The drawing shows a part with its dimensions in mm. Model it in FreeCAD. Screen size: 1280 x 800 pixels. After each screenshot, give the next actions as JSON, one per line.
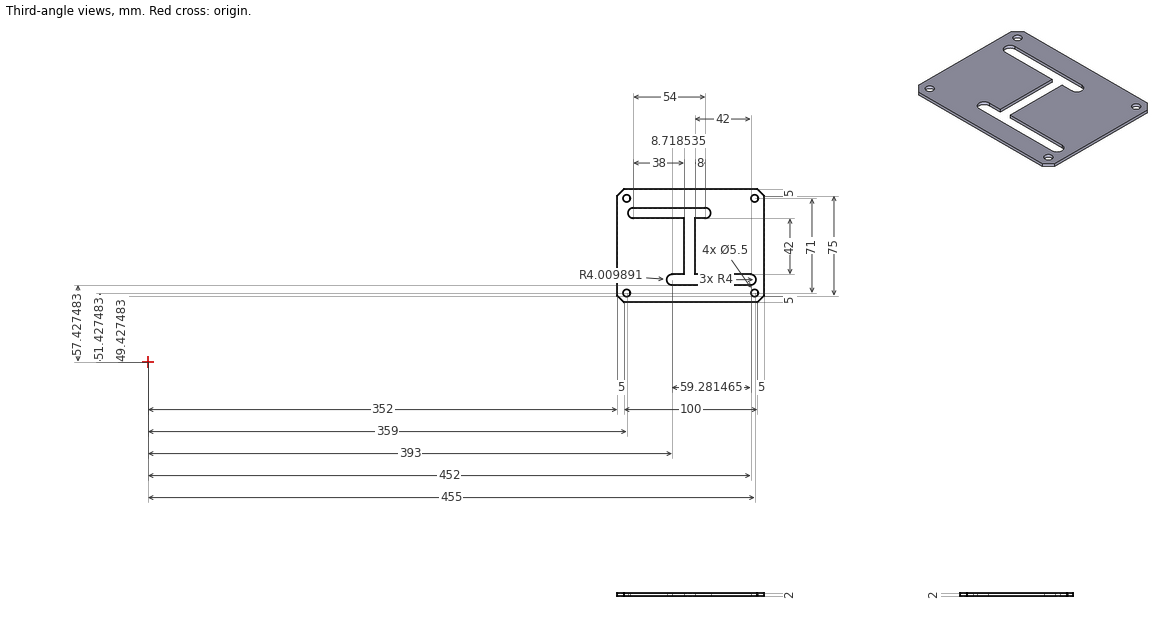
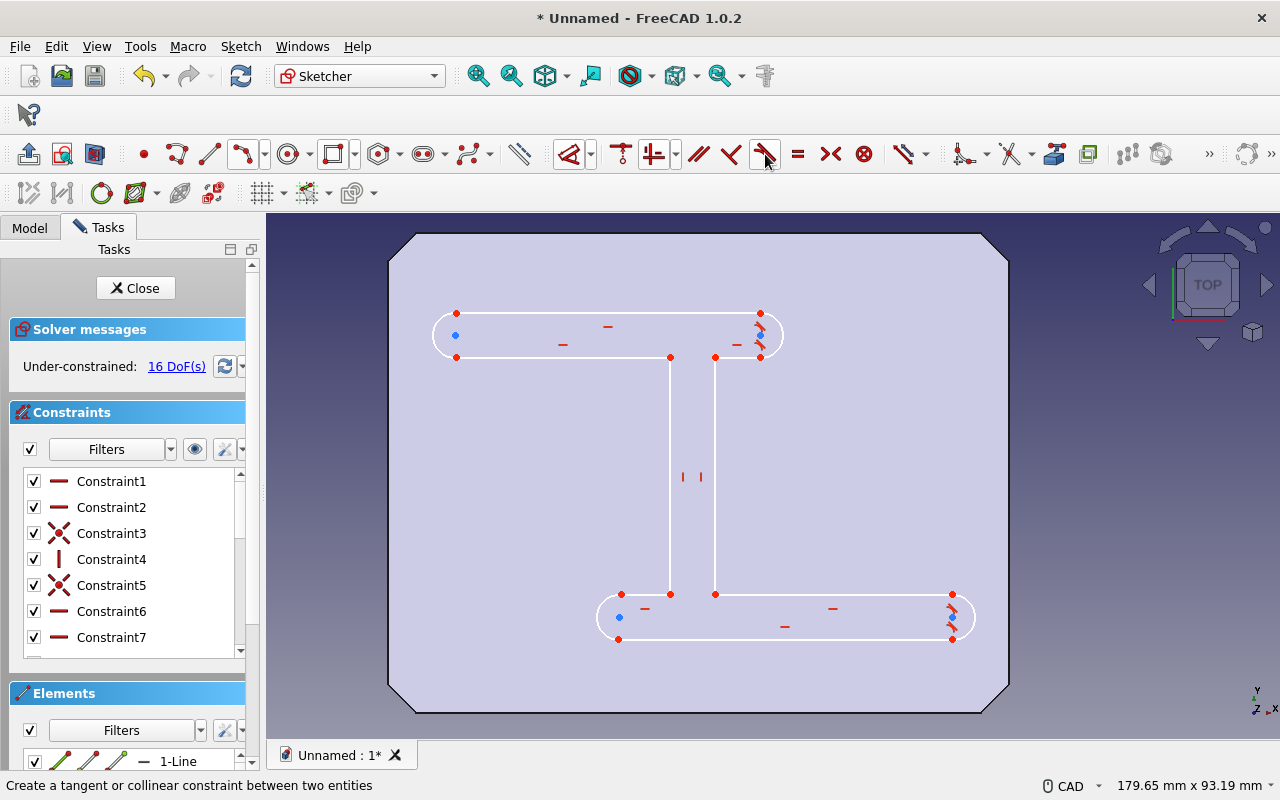
{"action": "left_click", "coordinate": [669, 313]}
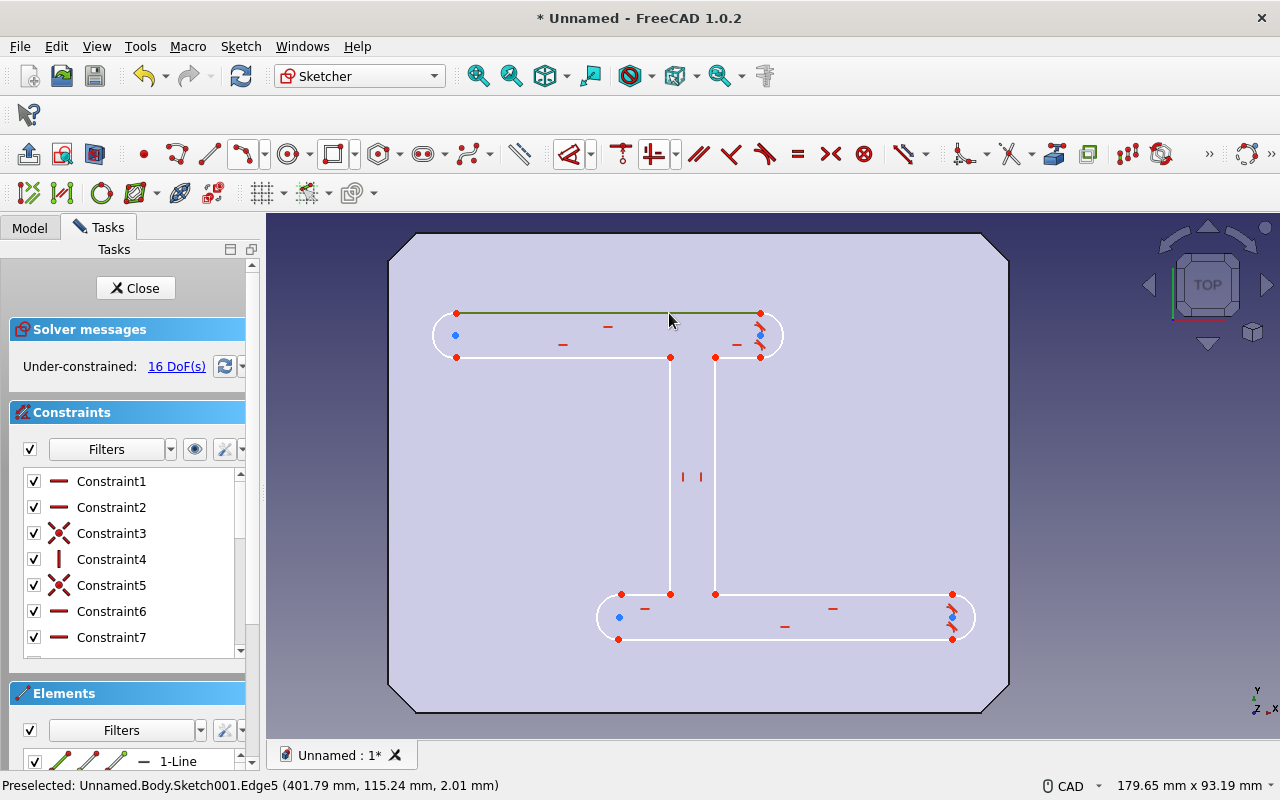
{"action": "left_click", "coordinate": [437, 322]}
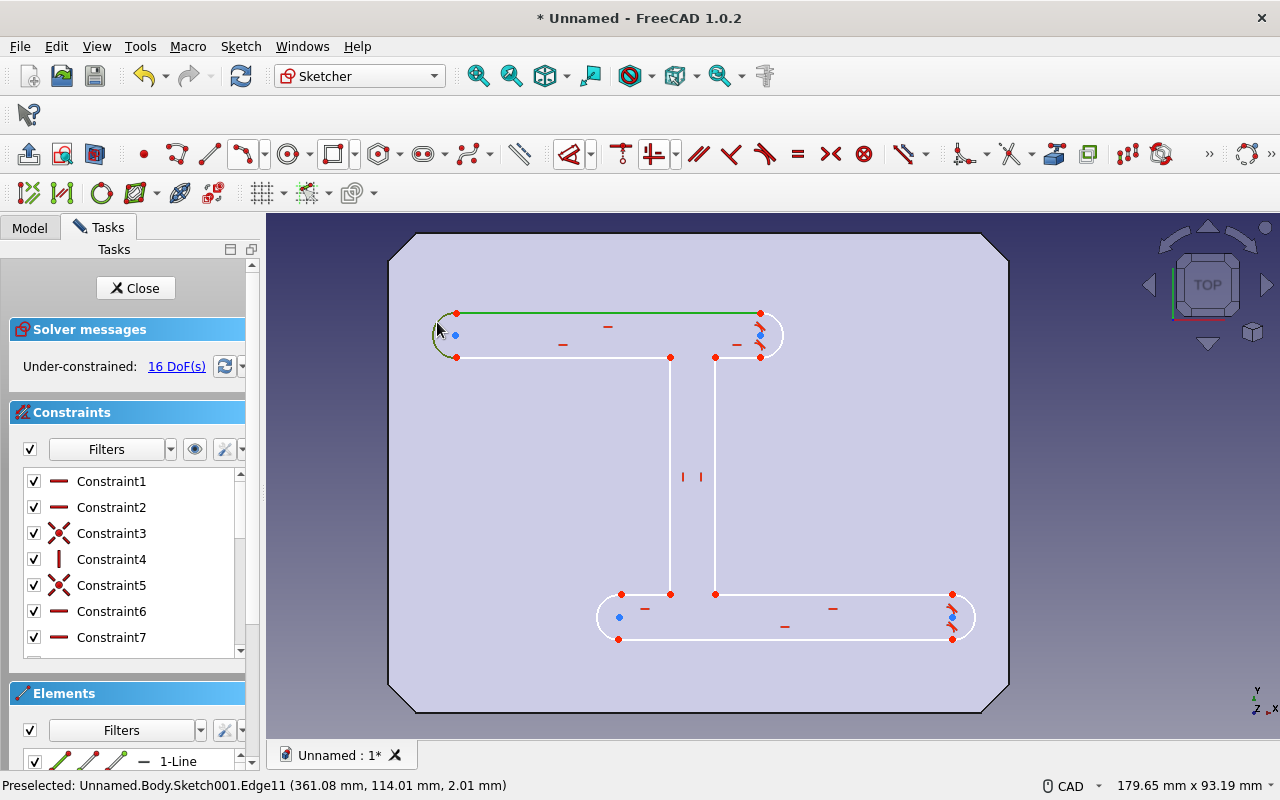
{"action": "left_click", "coordinate": [765, 154]}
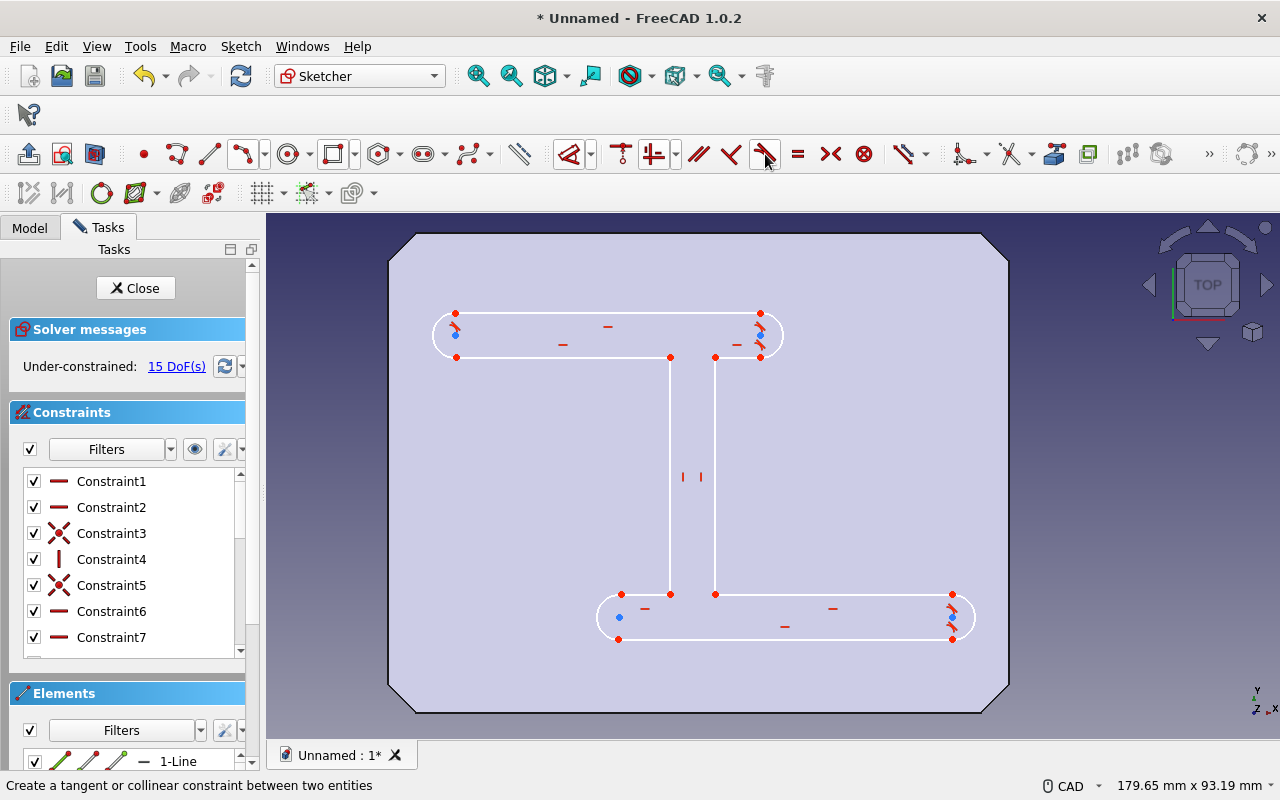
{"action": "left_click", "coordinate": [520, 358]}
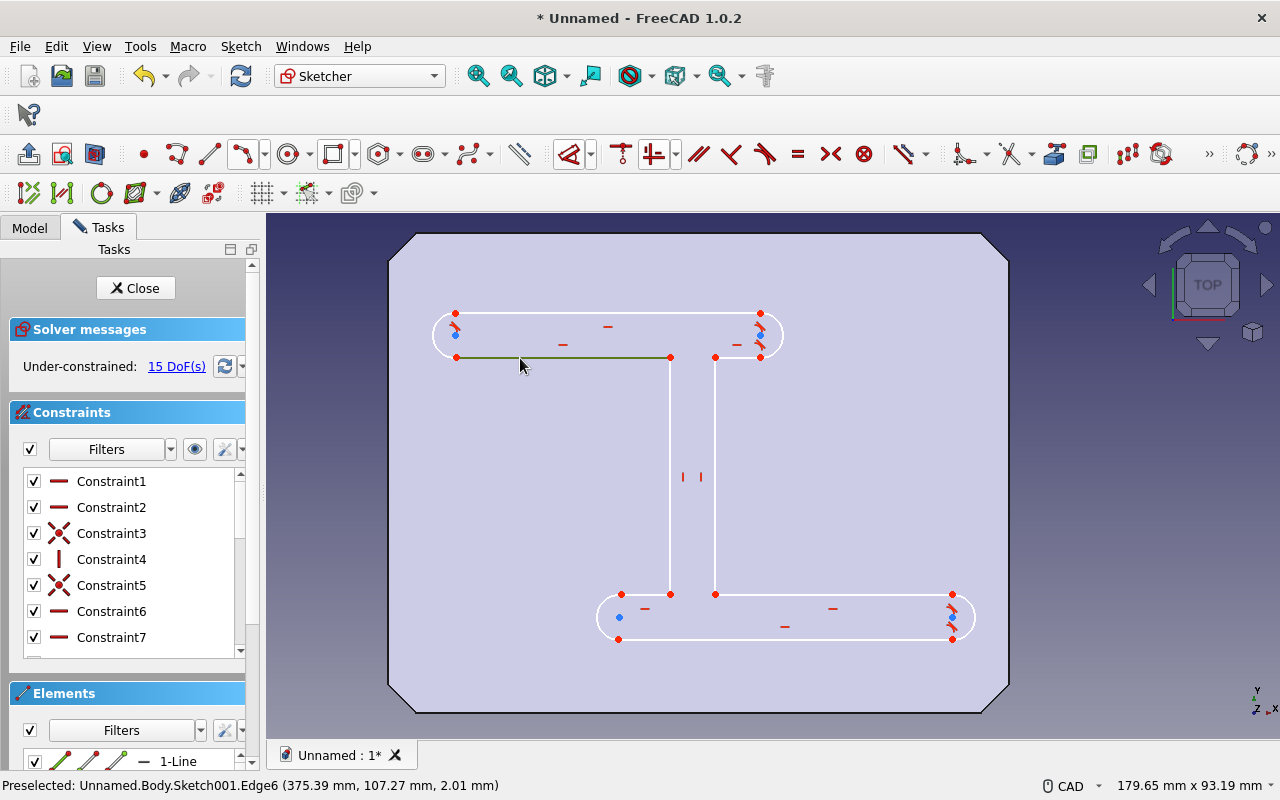
{"action": "left_click", "coordinate": [437, 322]}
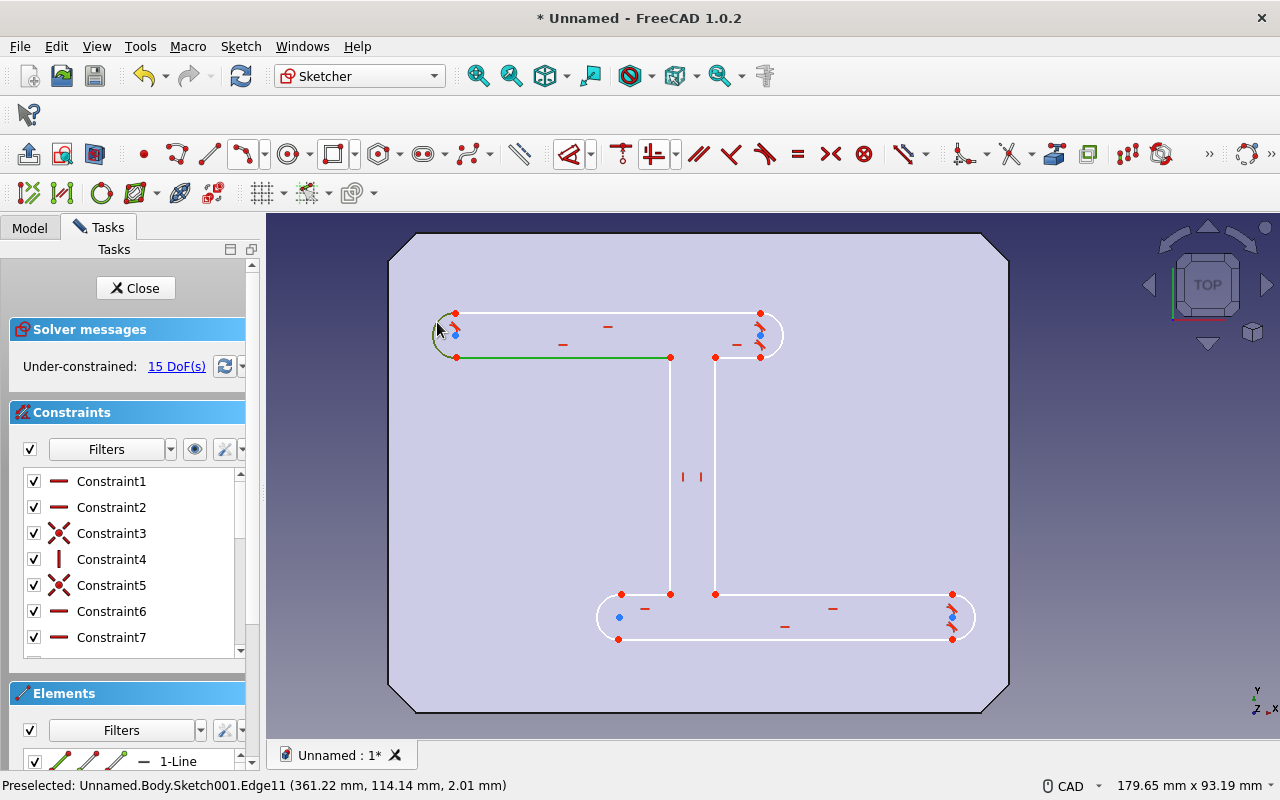
{"action": "left_click", "coordinate": [765, 154]}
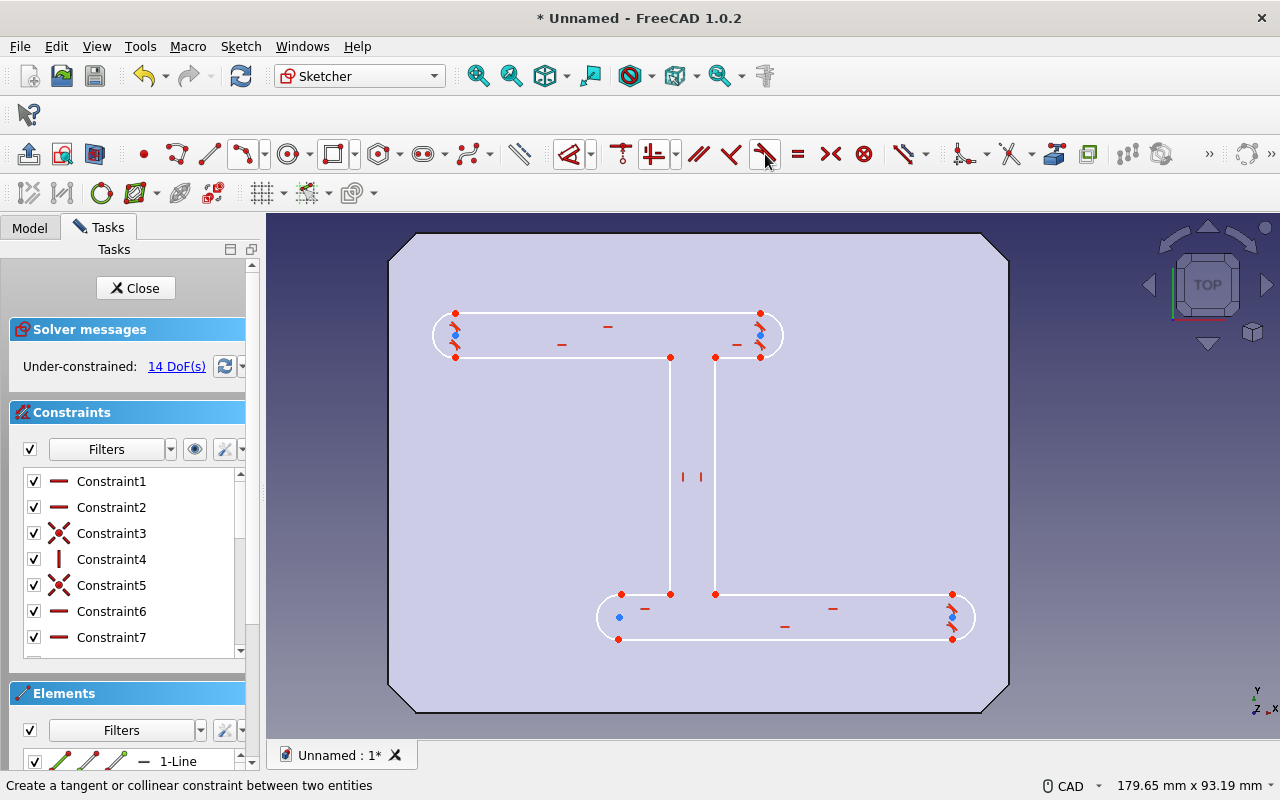
{"action": "left_click", "coordinate": [971, 631]}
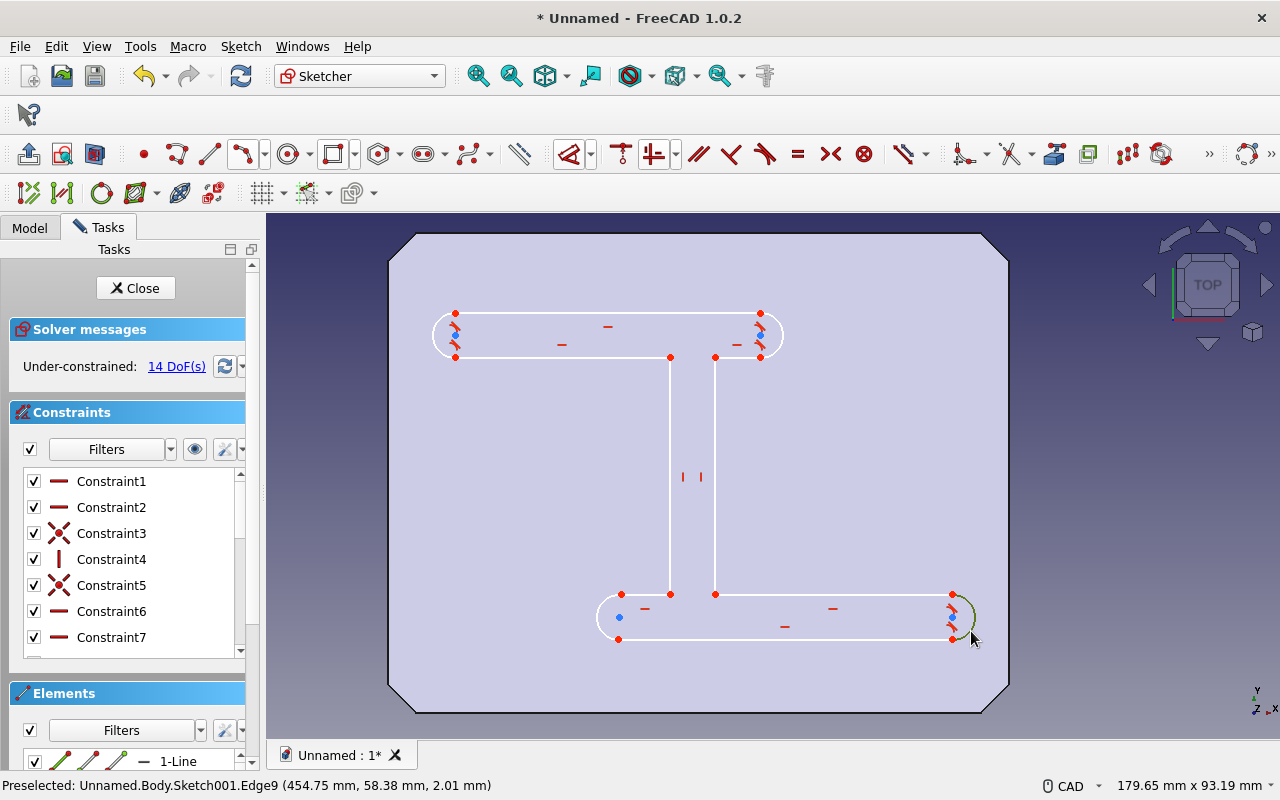
{"action": "left_click", "coordinate": [779, 349]}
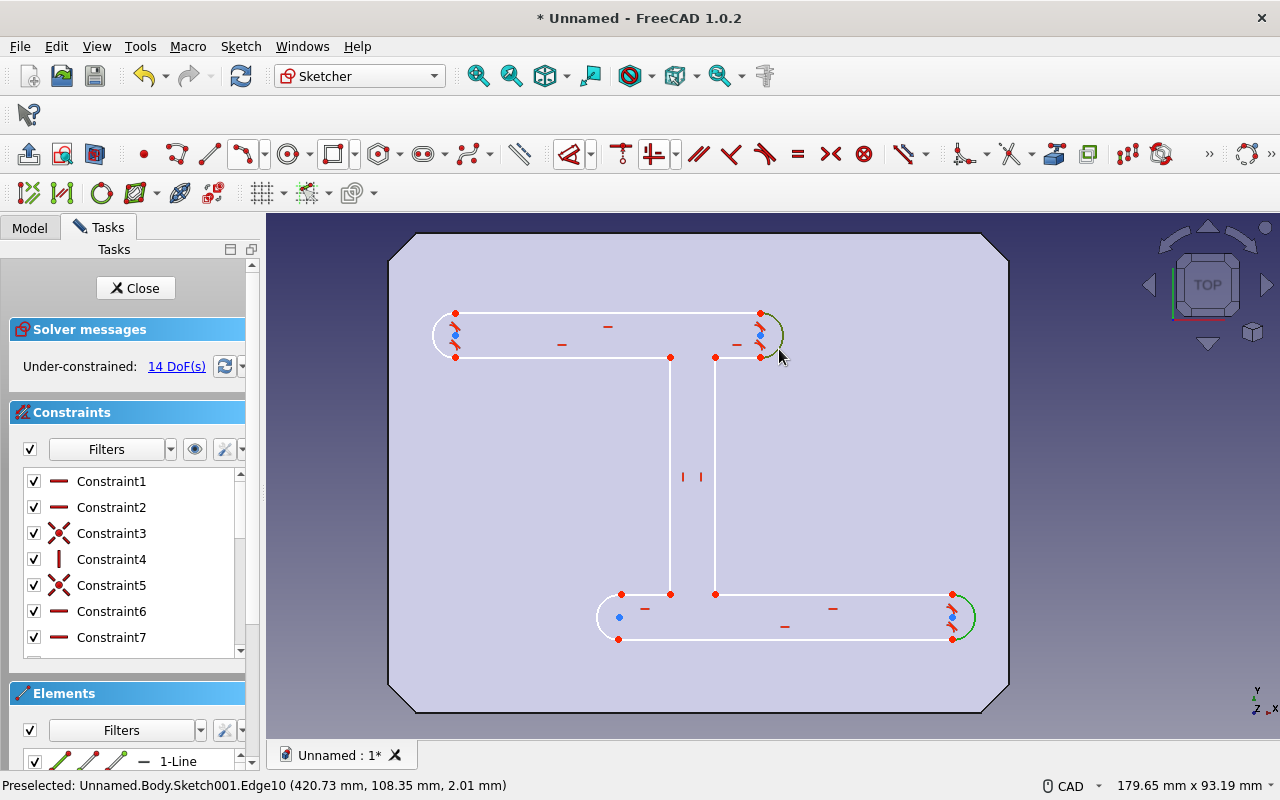
{"action": "left_click", "coordinate": [437, 322]}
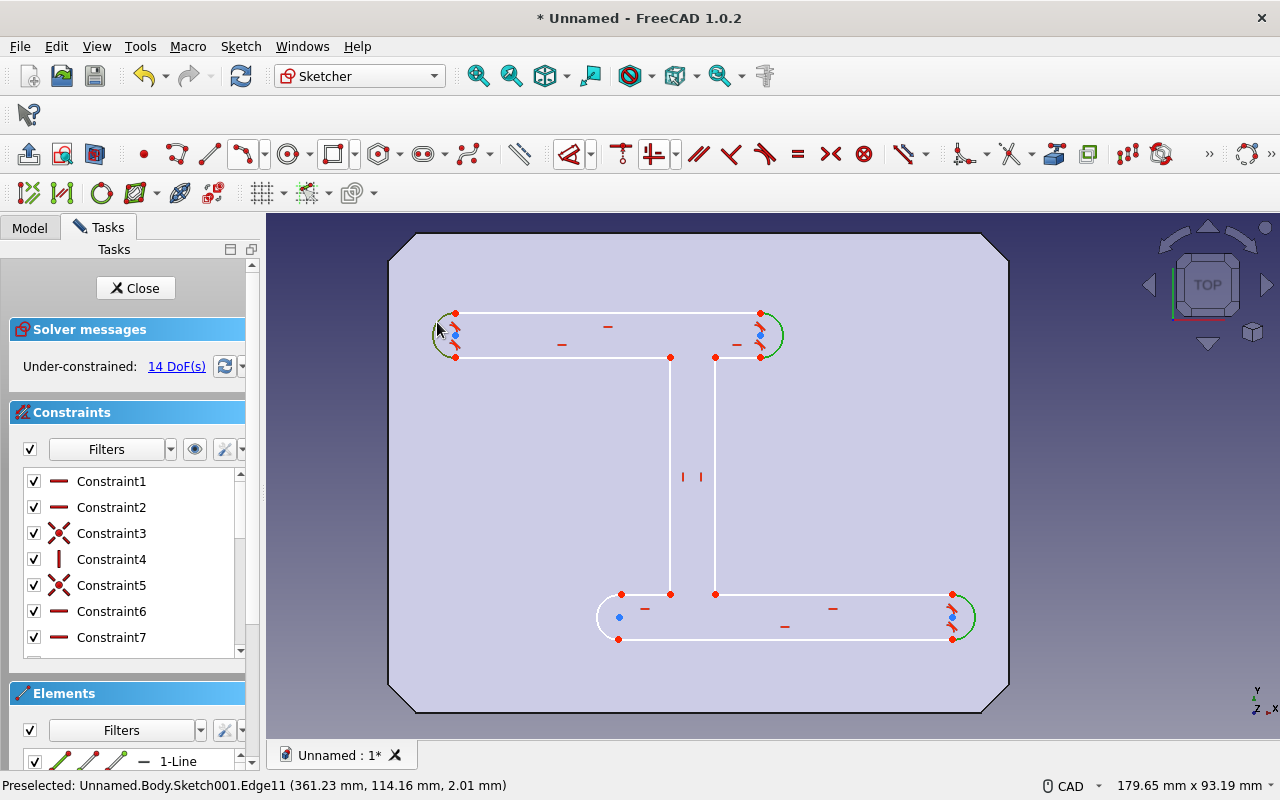
{"action": "left_click", "coordinate": [798, 154]}